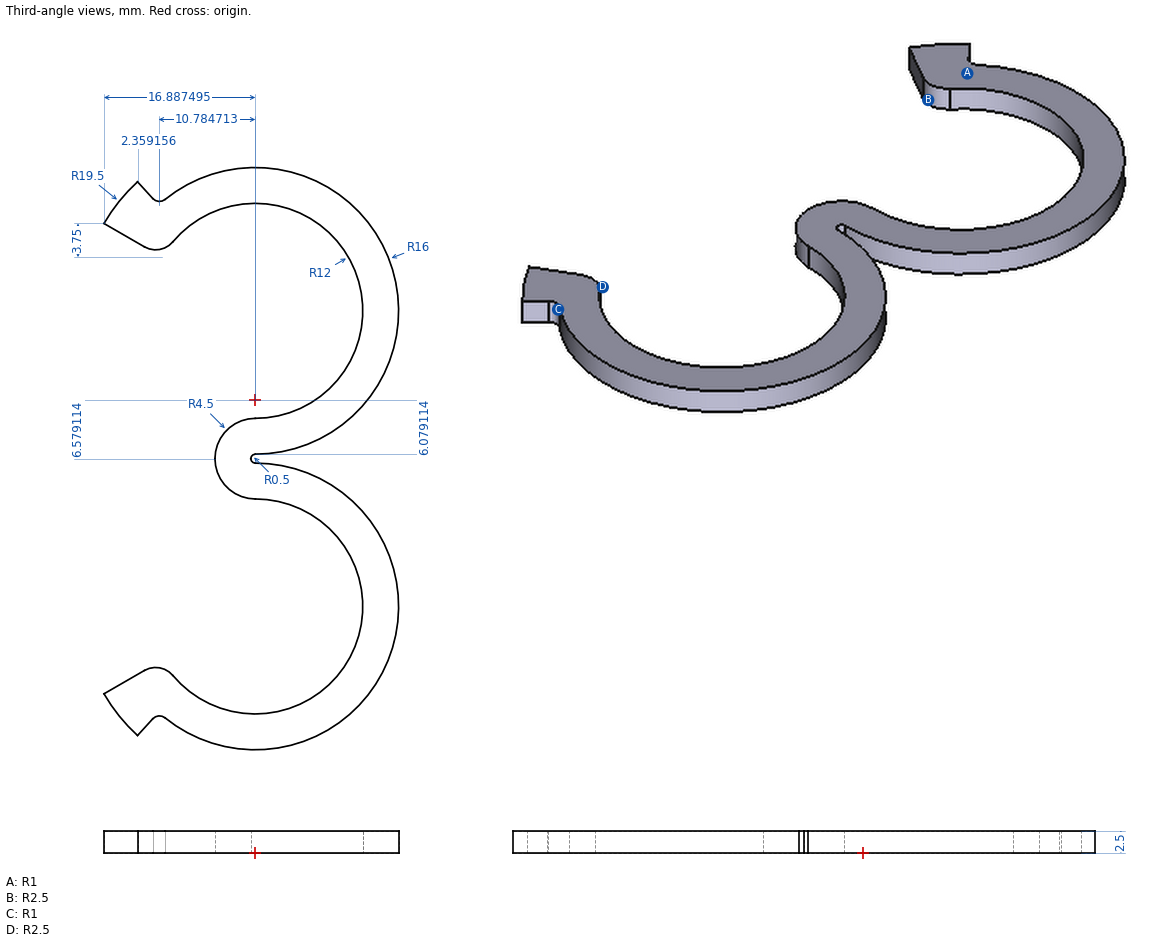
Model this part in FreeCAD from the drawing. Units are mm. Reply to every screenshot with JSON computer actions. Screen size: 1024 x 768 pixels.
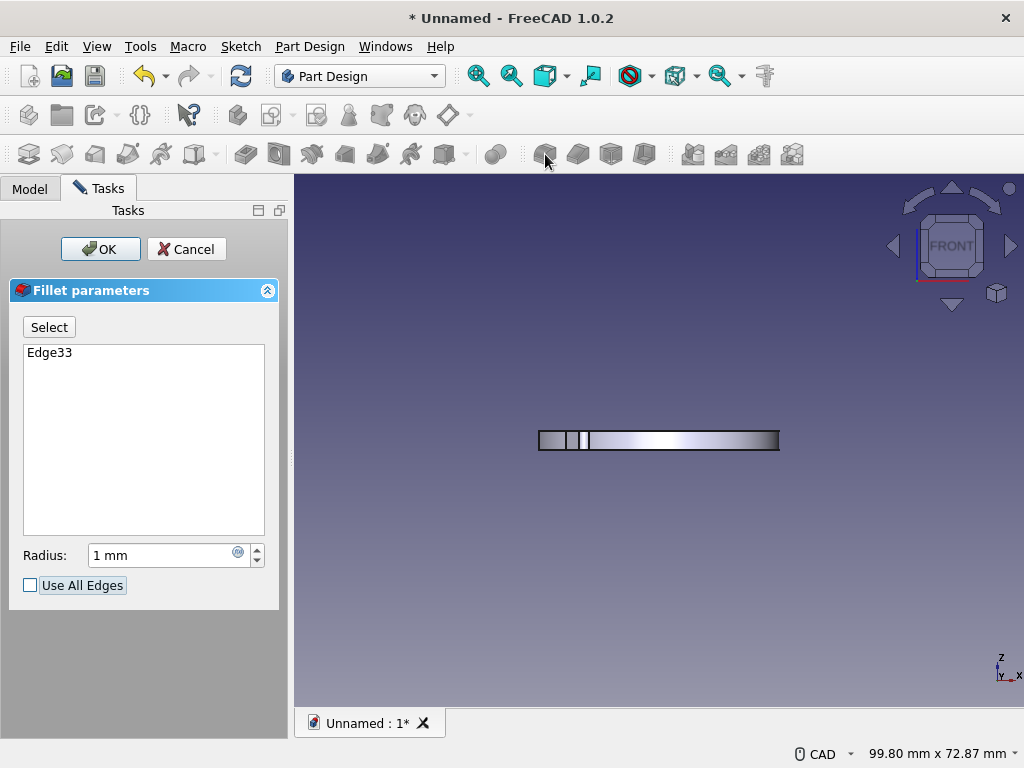
{"action": "left_click", "coordinate": [101, 249]}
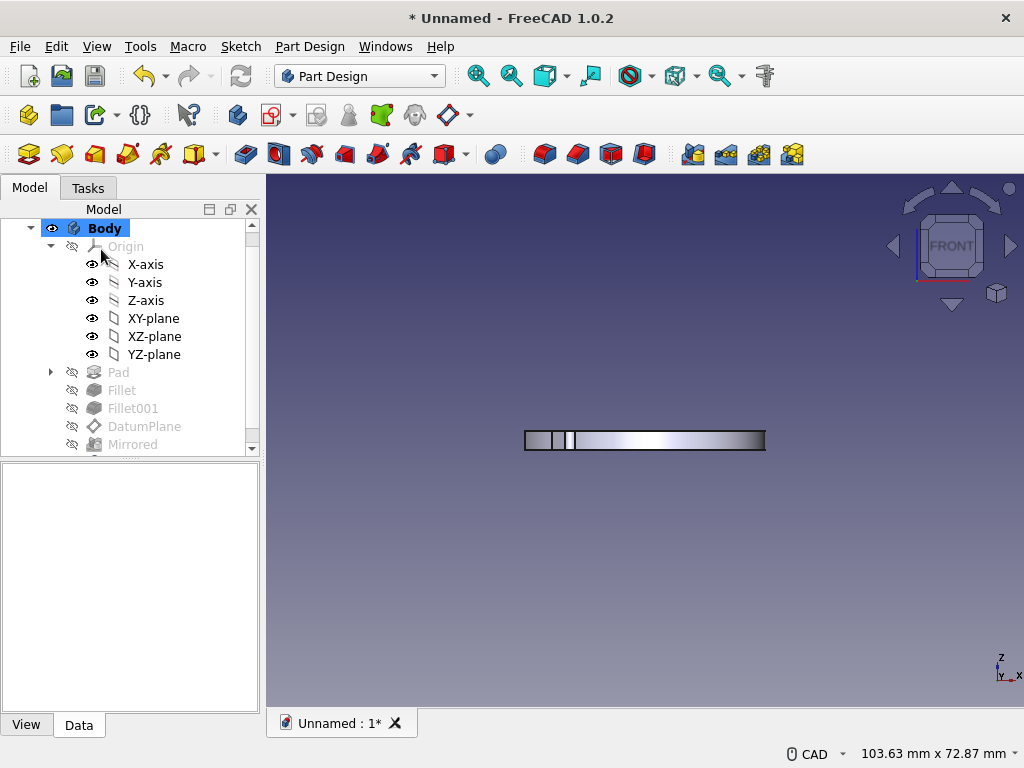
{"action": "left_click", "coordinate": [479, 76]}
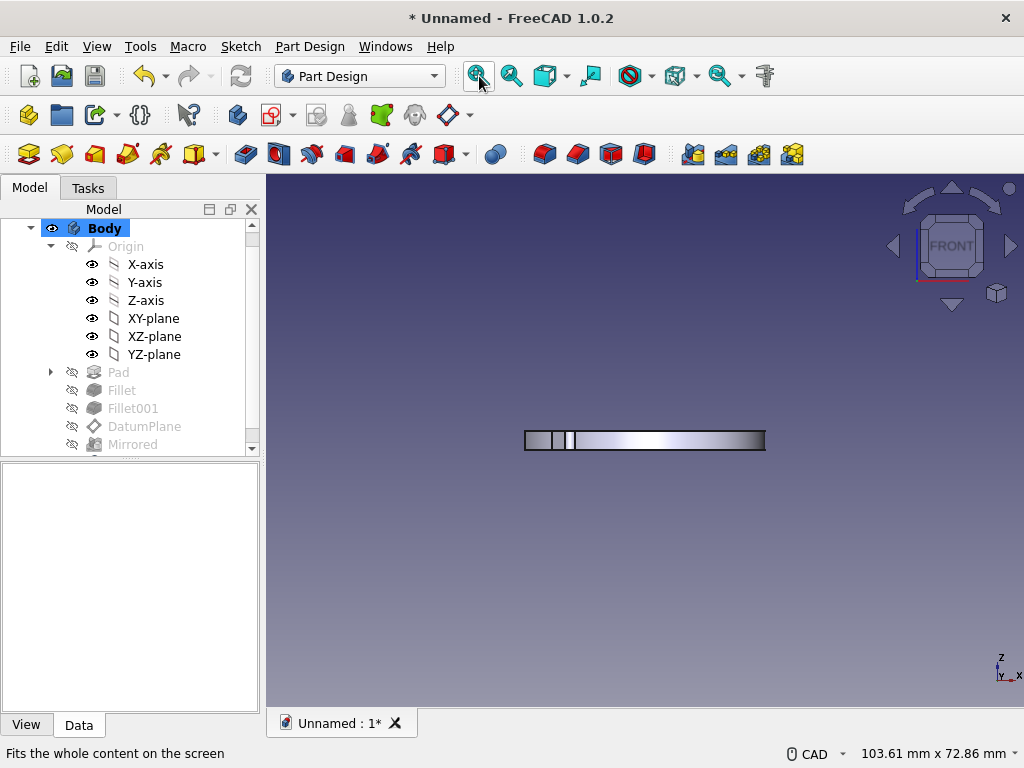
{"action": "scroll", "coordinate": [572, 440], "scroll_direction": "up", "scroll_amount": 4}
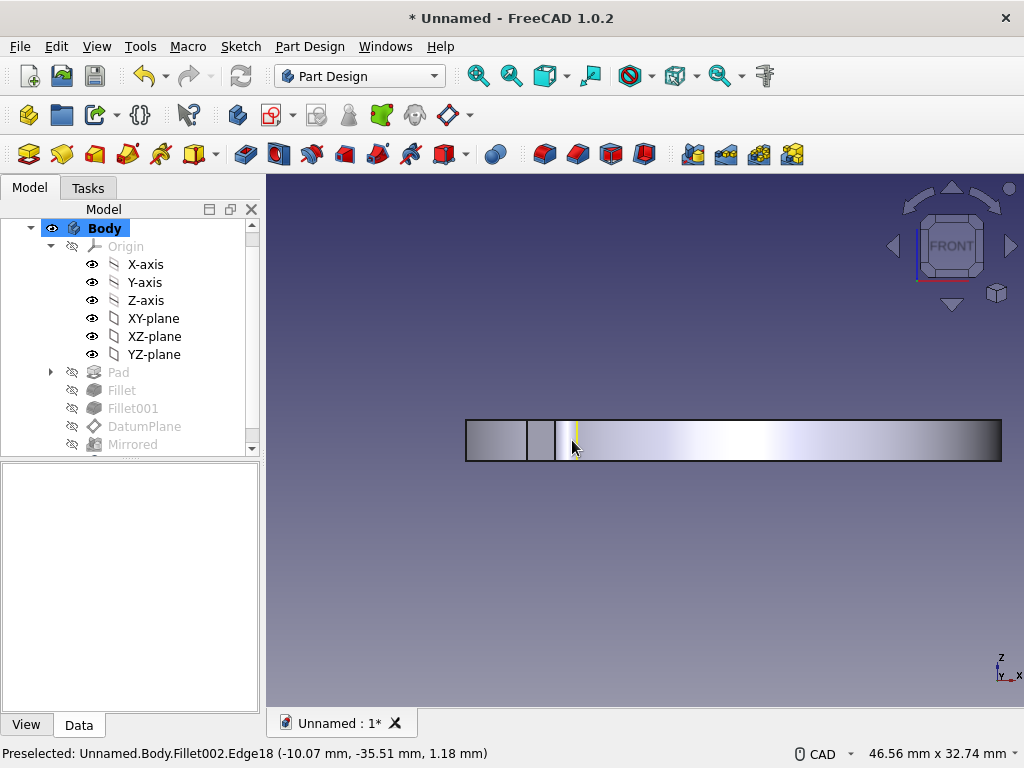
{"action": "left_click", "coordinate": [479, 76]}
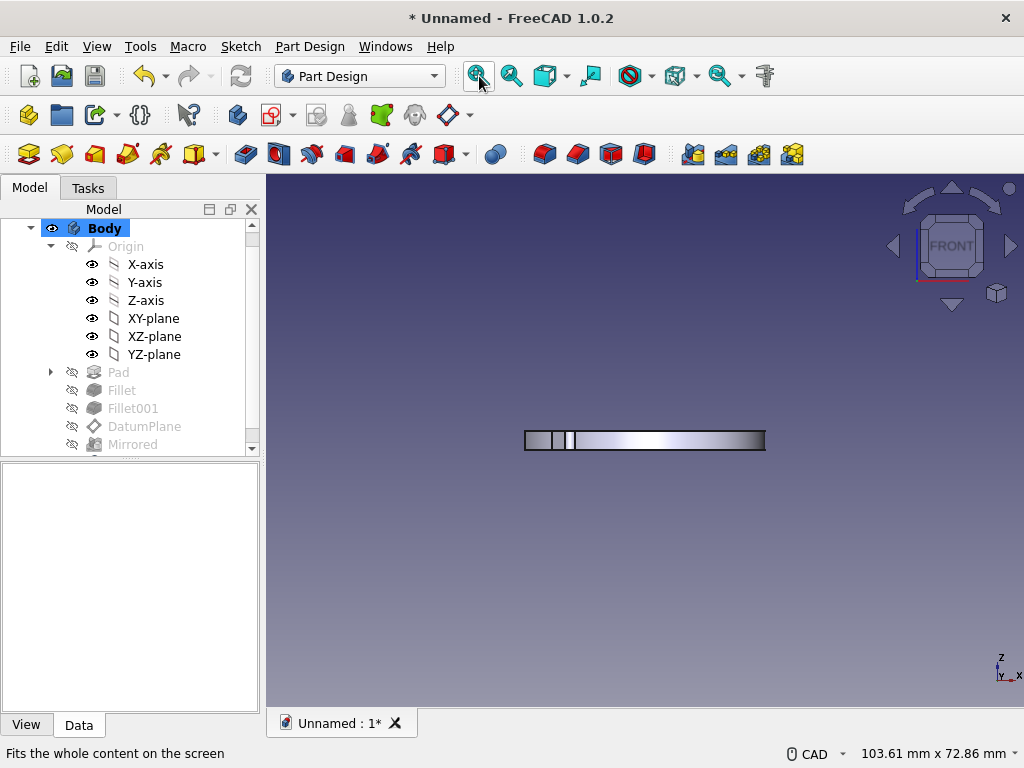
{"action": "key", "text": "0"}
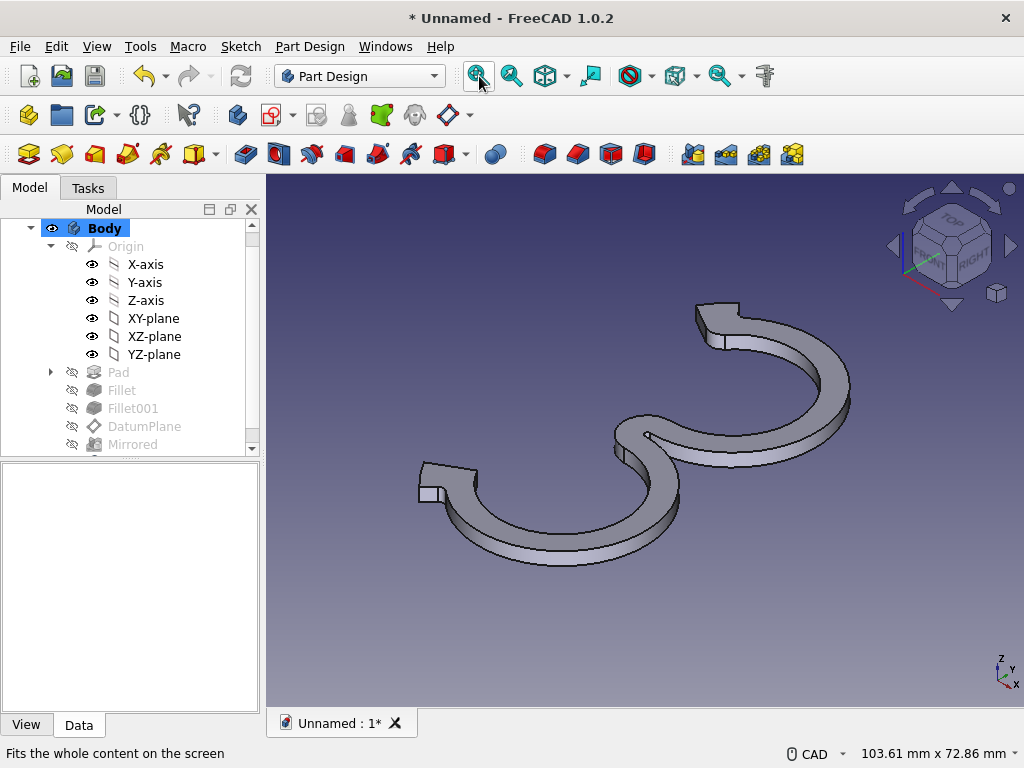
{"action": "scroll", "coordinate": [477, 477], "scroll_direction": "up", "scroll_amount": 4}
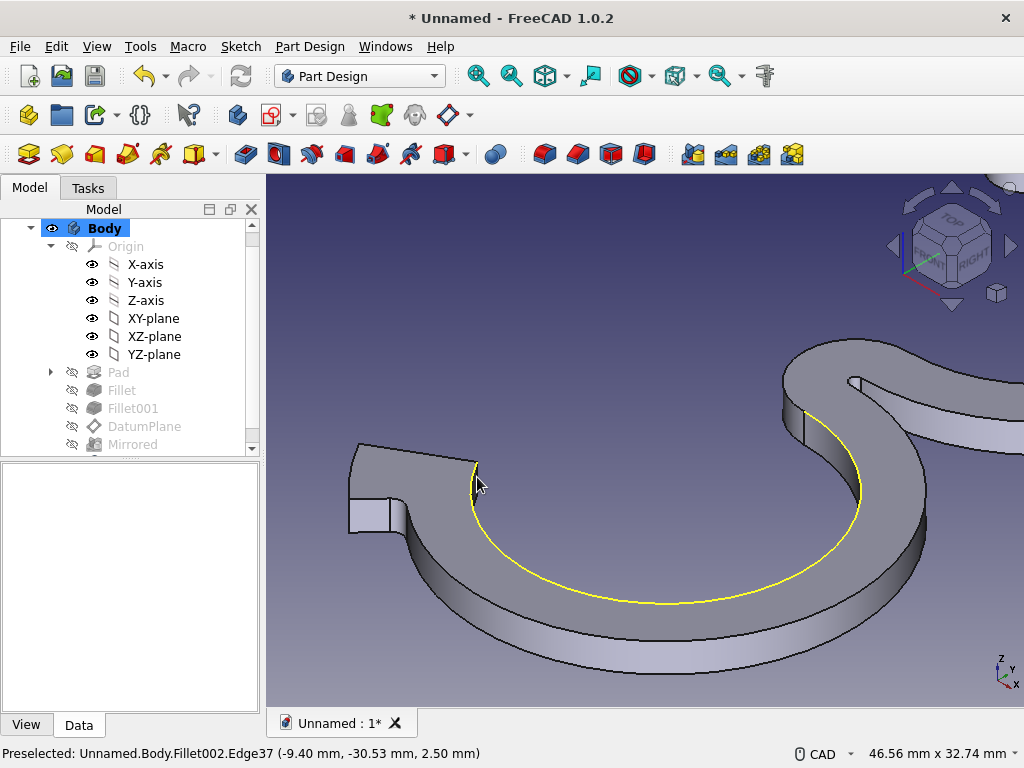
{"action": "left_click", "coordinate": [479, 76]}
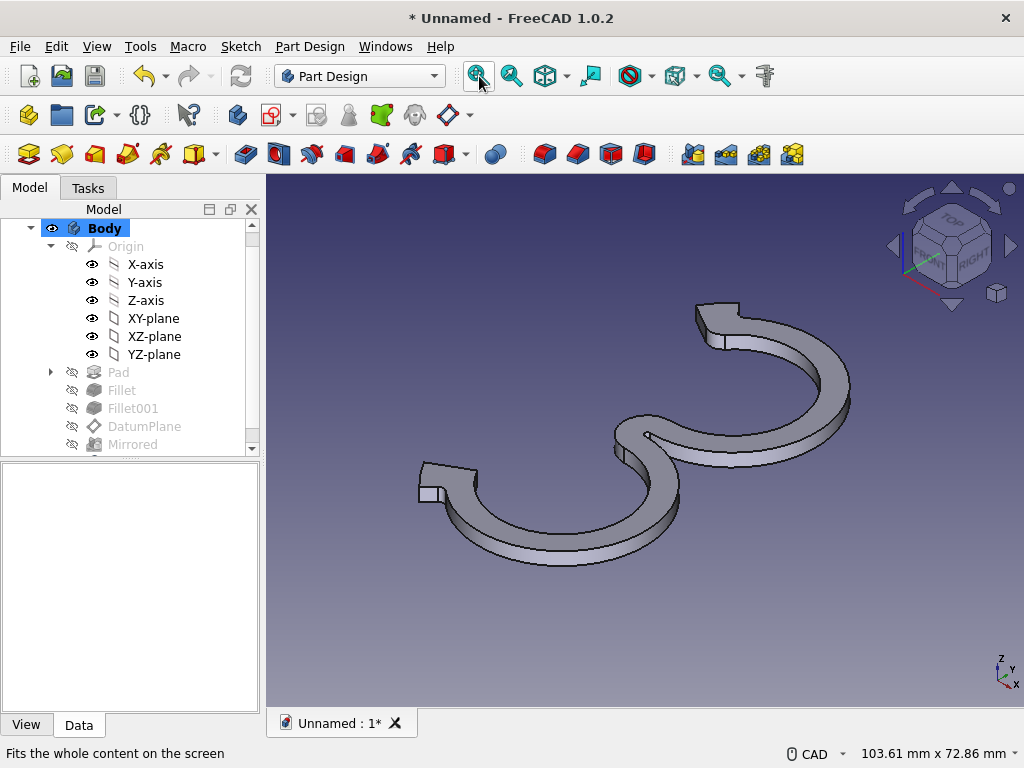
{"action": "key", "text": "2"}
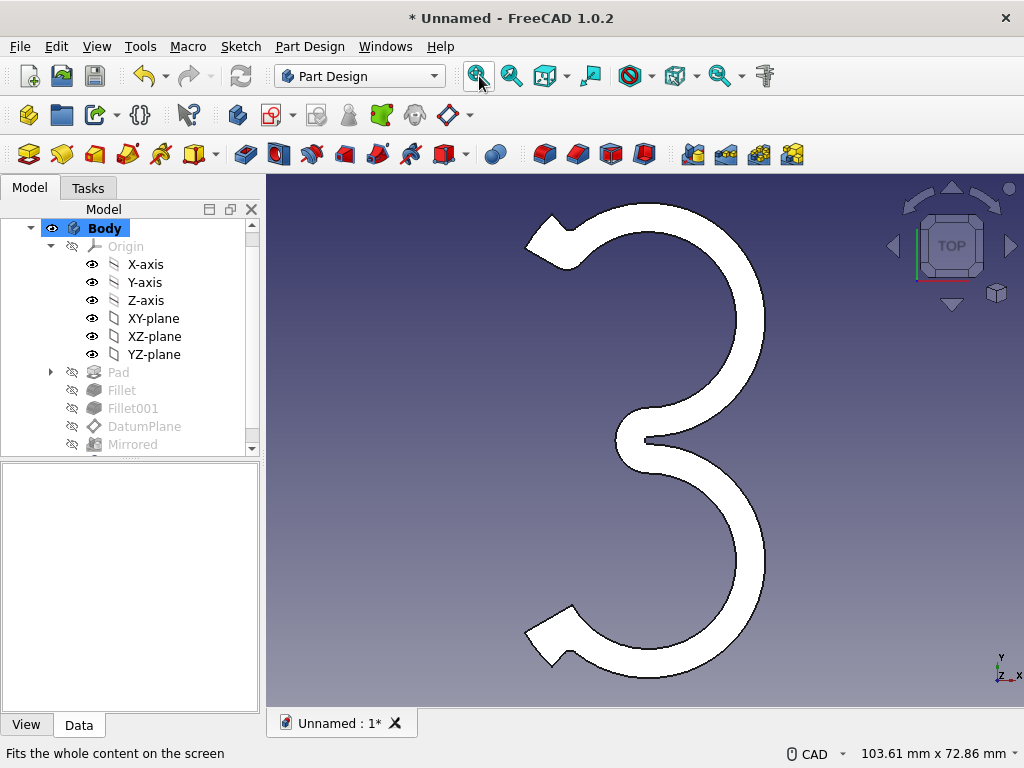
{"action": "scroll", "coordinate": [572, 604], "scroll_direction": "up", "scroll_amount": 4}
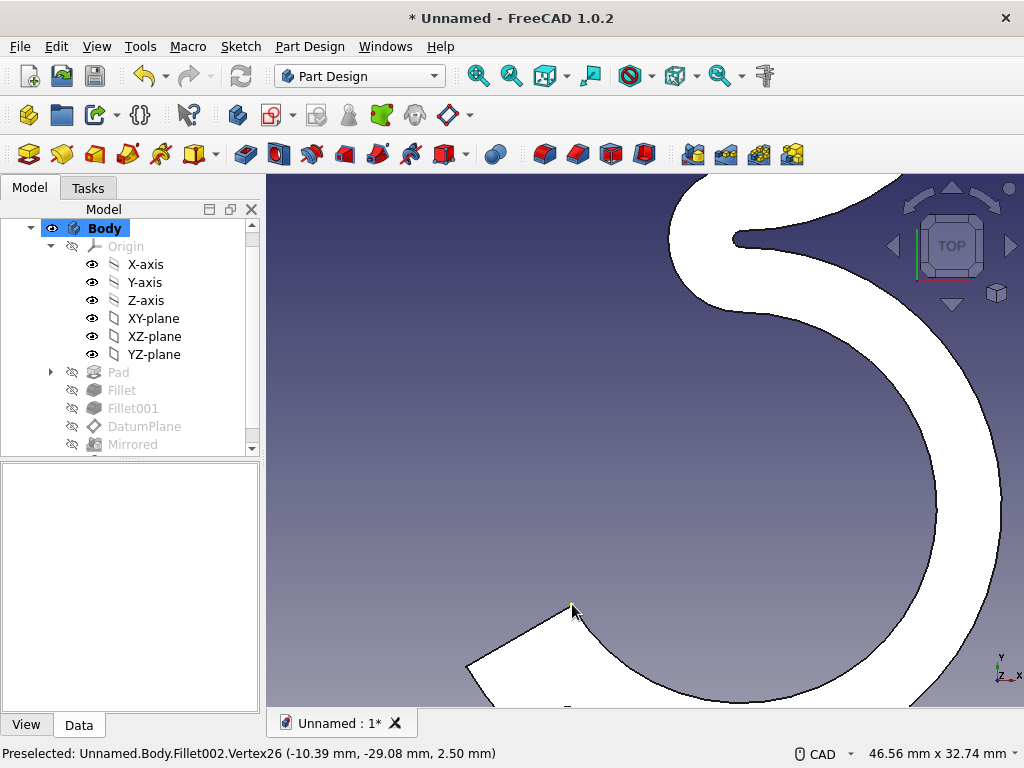
{"action": "left_click", "coordinate": [479, 76]}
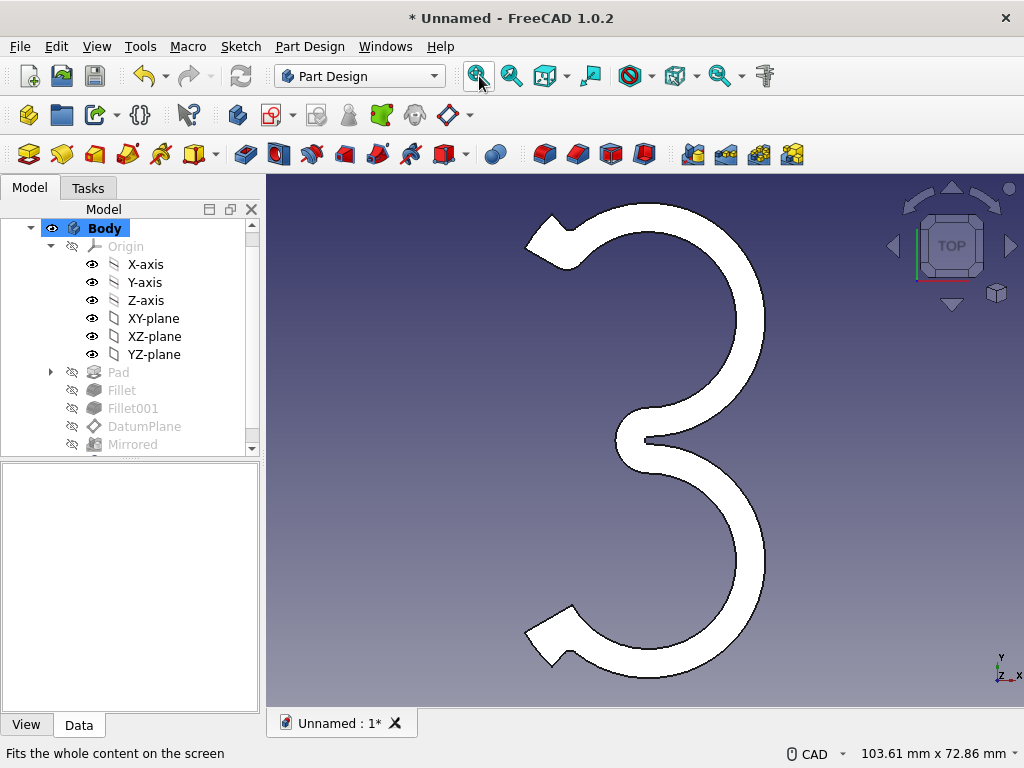
{"action": "key", "text": "1"}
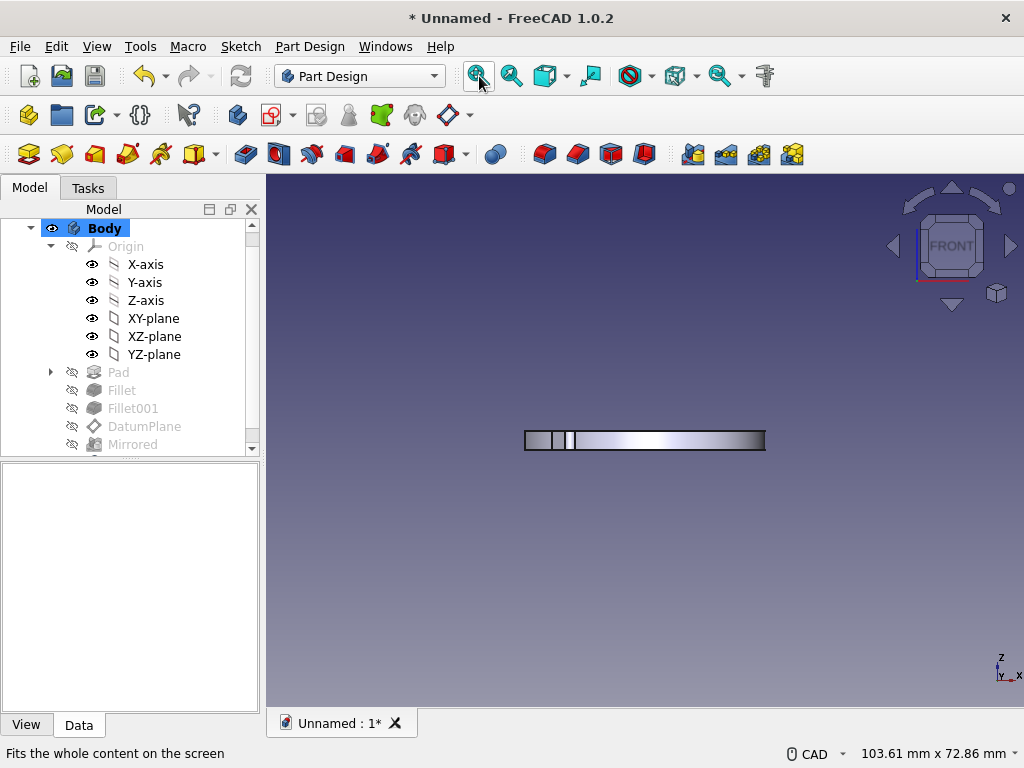
{"action": "left_click", "coordinate": [479, 76]}